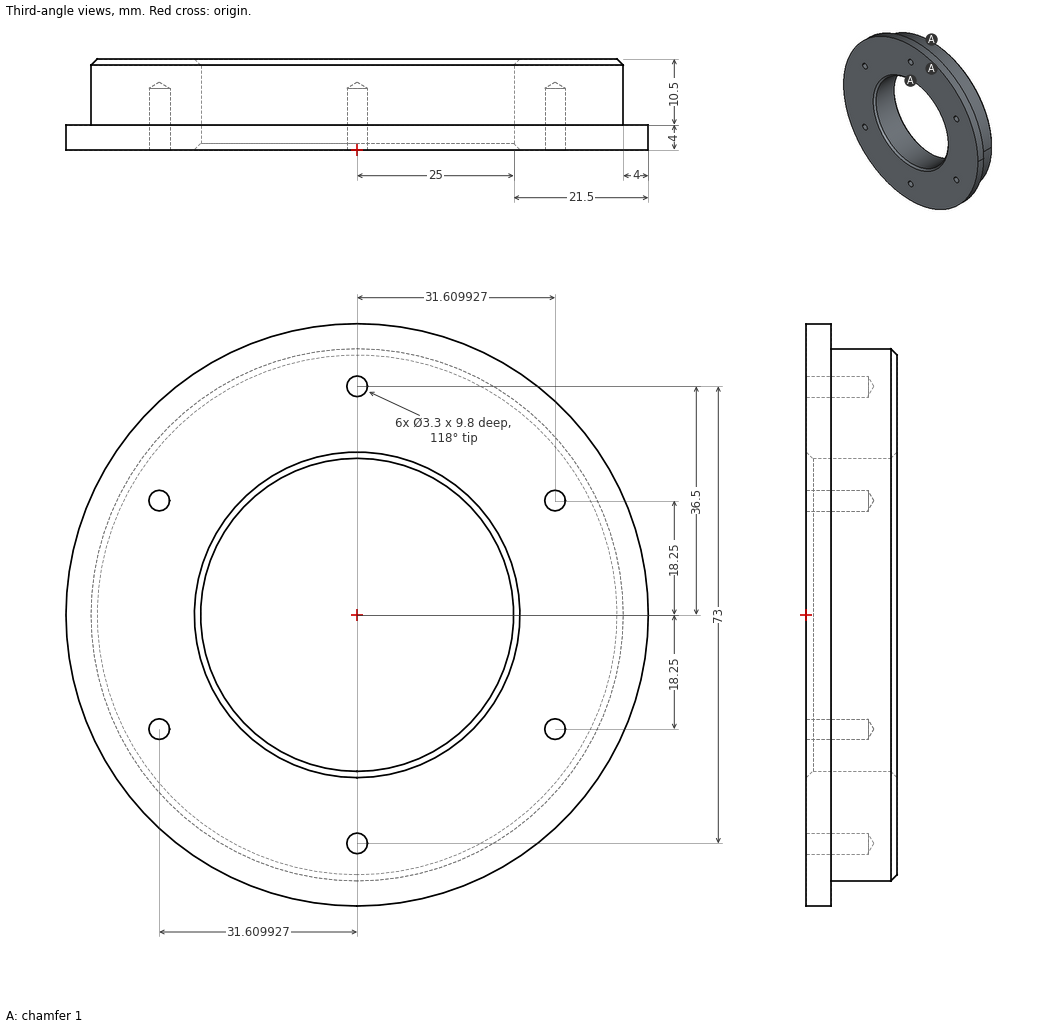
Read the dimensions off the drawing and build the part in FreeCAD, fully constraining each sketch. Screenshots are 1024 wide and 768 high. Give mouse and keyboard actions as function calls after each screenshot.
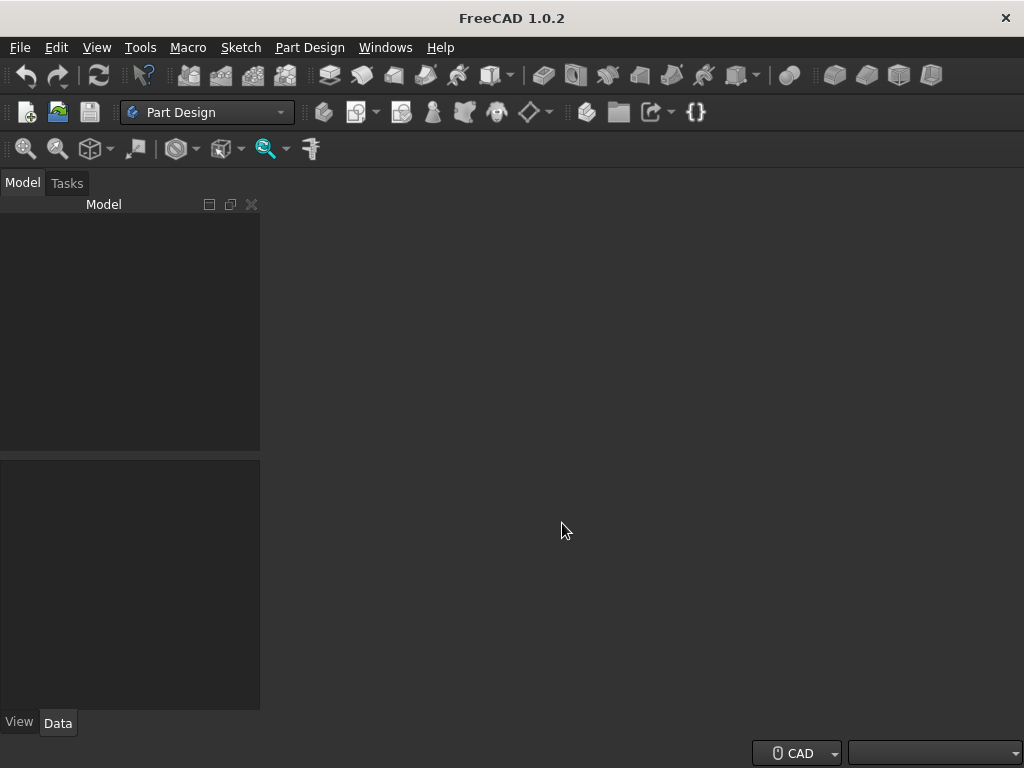
click(26, 112)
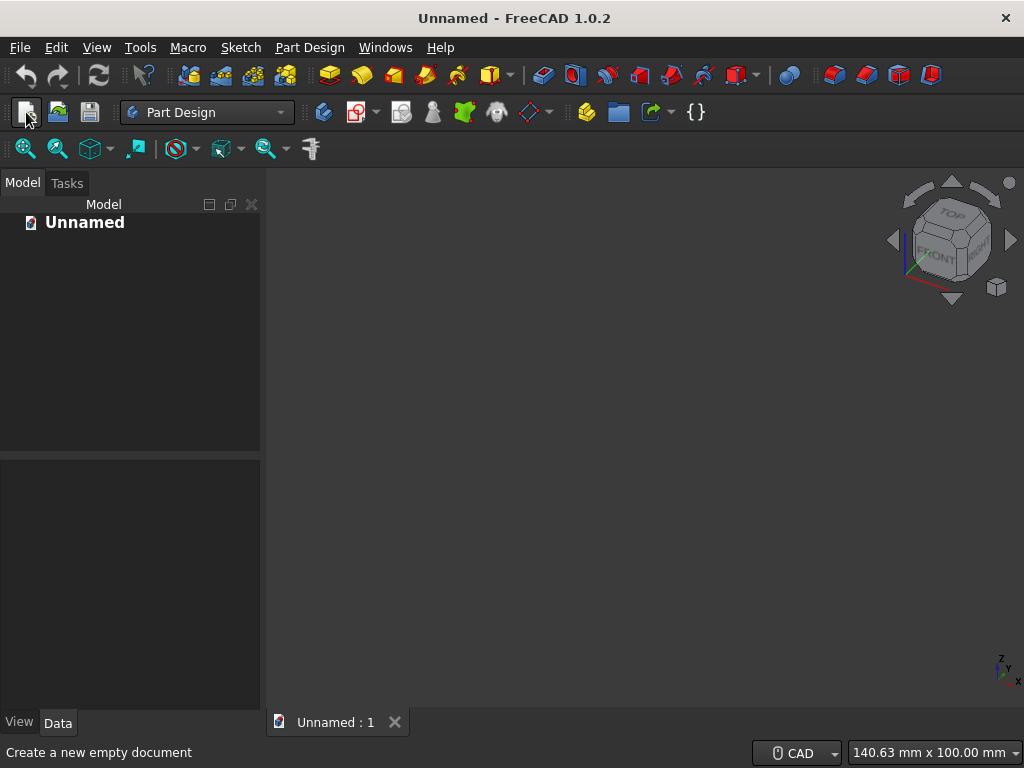
click(356, 112)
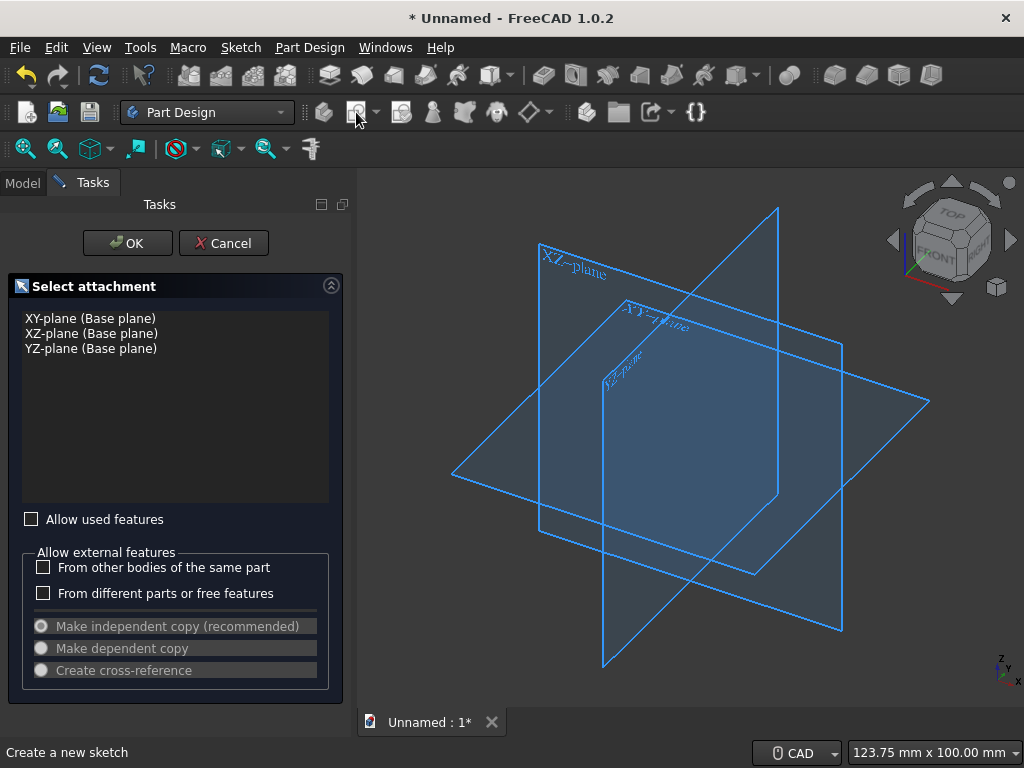
click(82, 318)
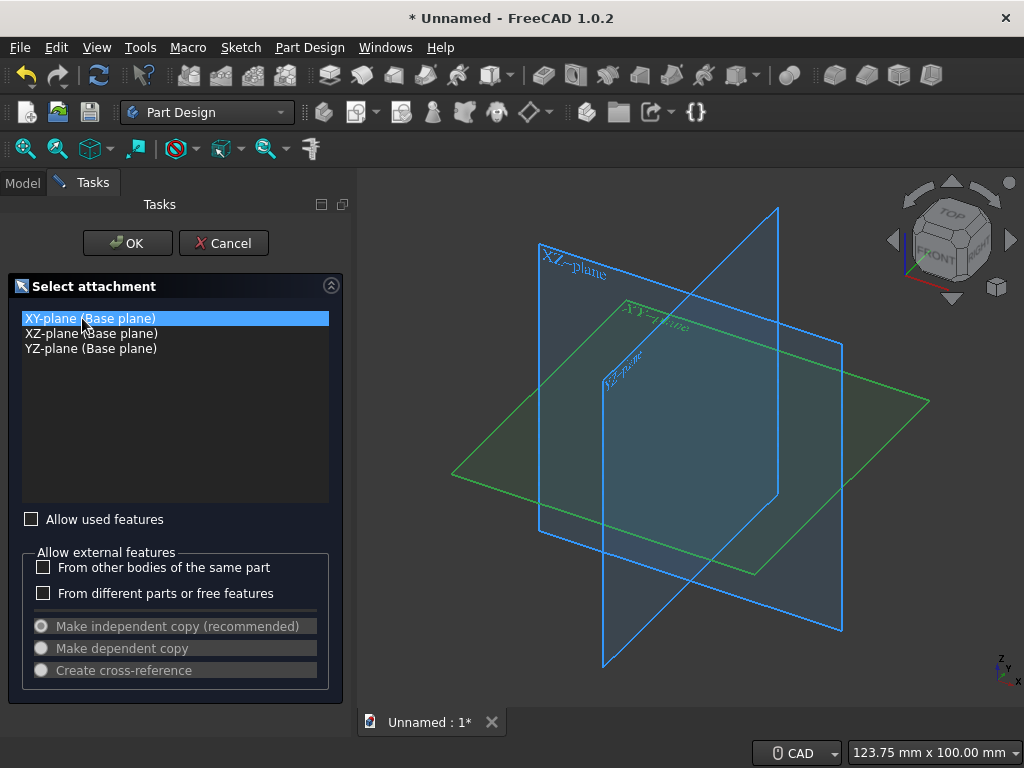
click(128, 243)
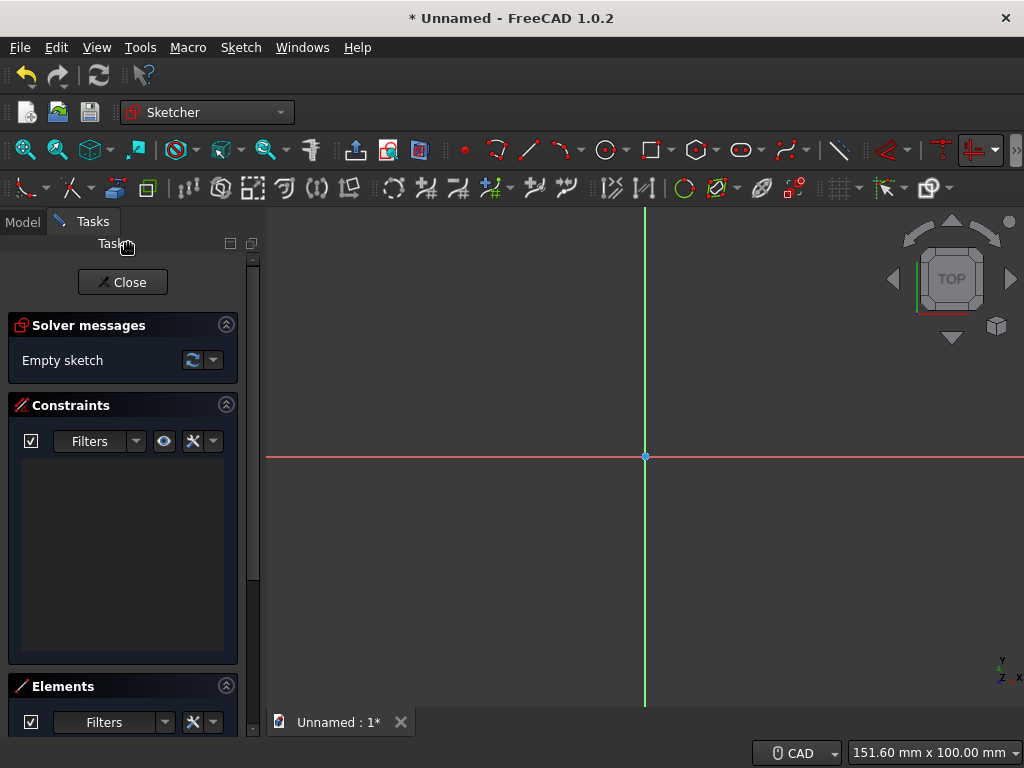
scroll(576, 457, down, 5)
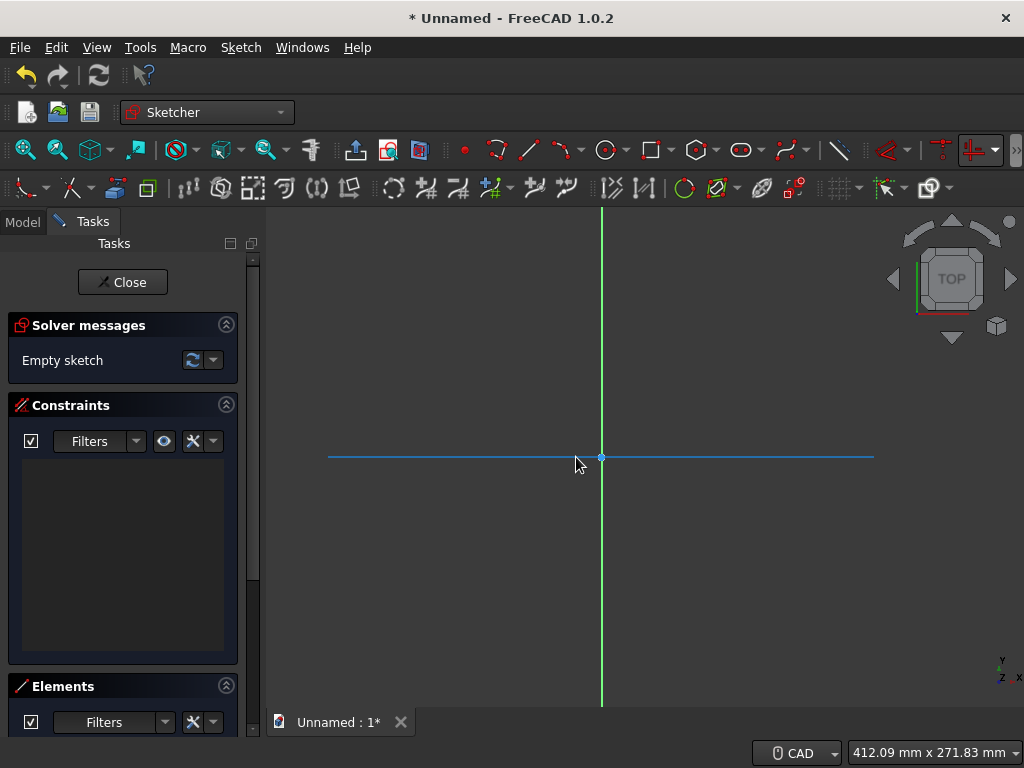
scroll(662, 441, up, 8)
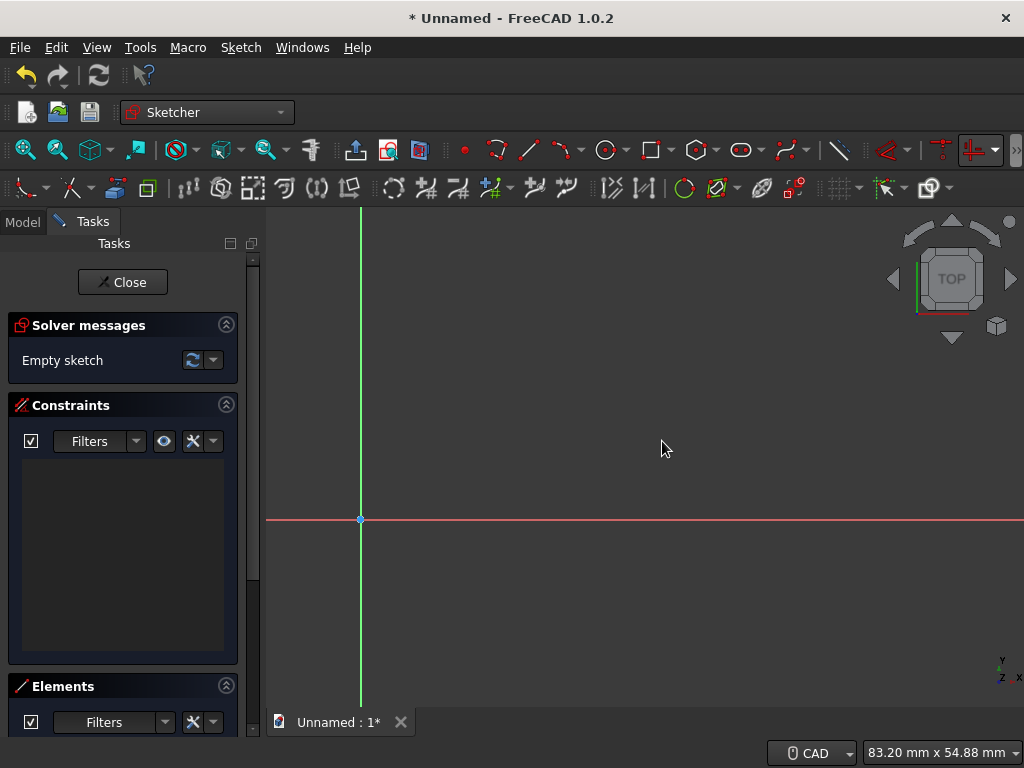
click(498, 150)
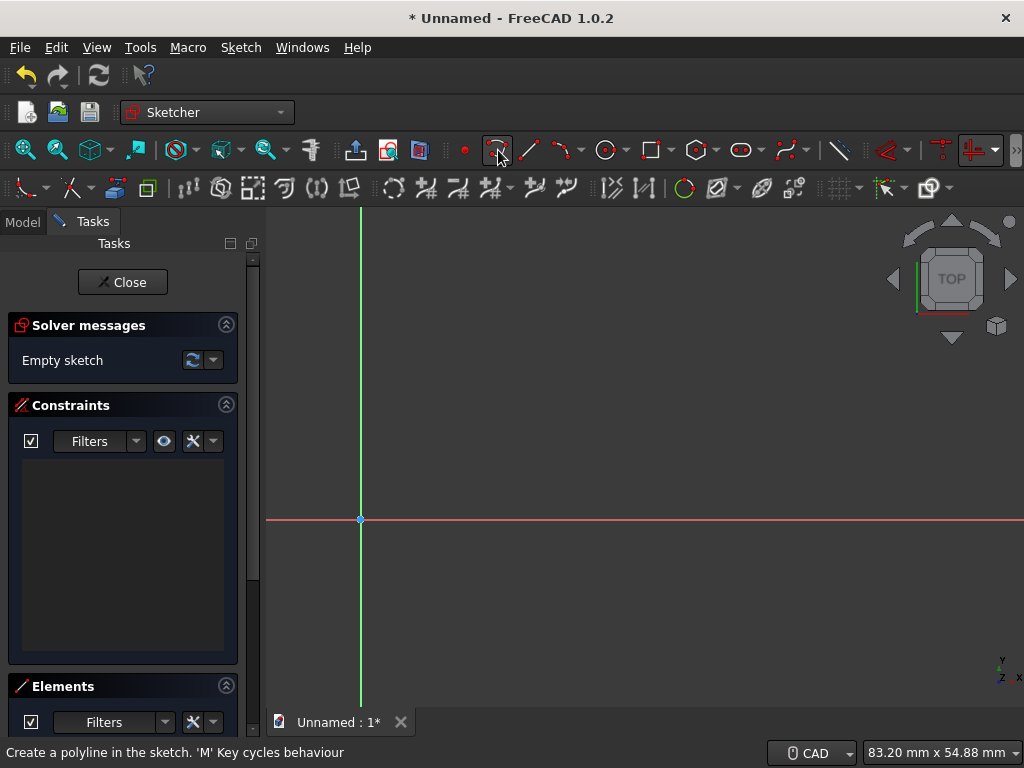
click(589, 520)
click(785, 511)
click(785, 484)
click(748, 484)
click(748, 388)
click(589, 388)
click(589, 520)
key(Escape)
key(Escape)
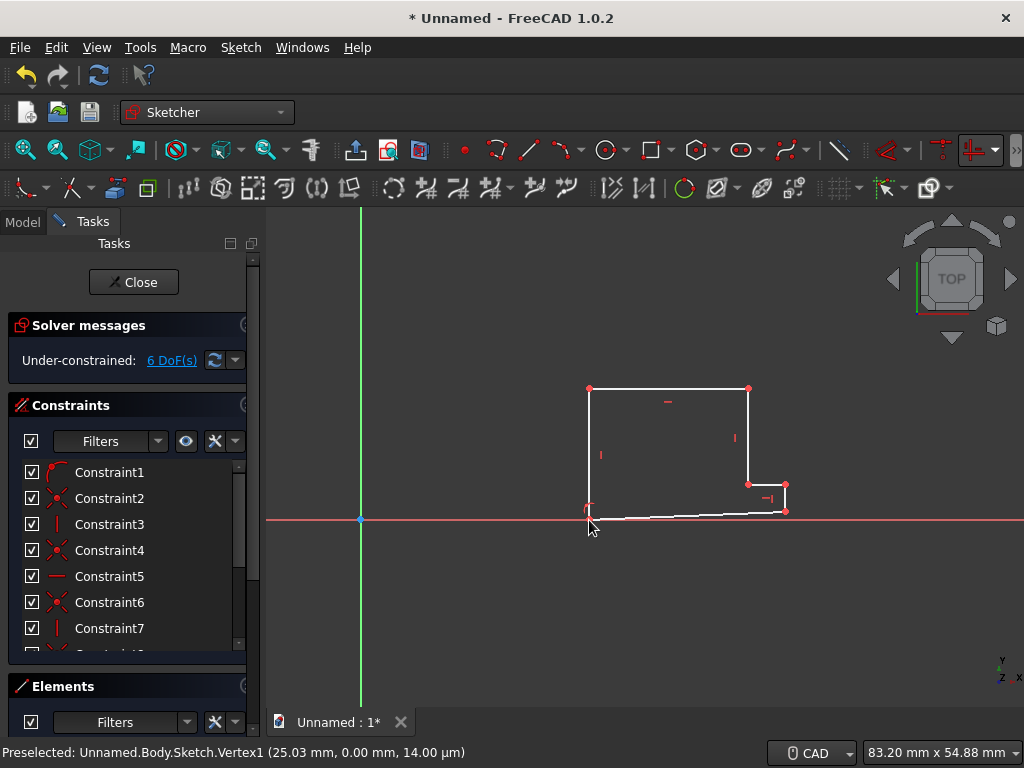
click(648, 518)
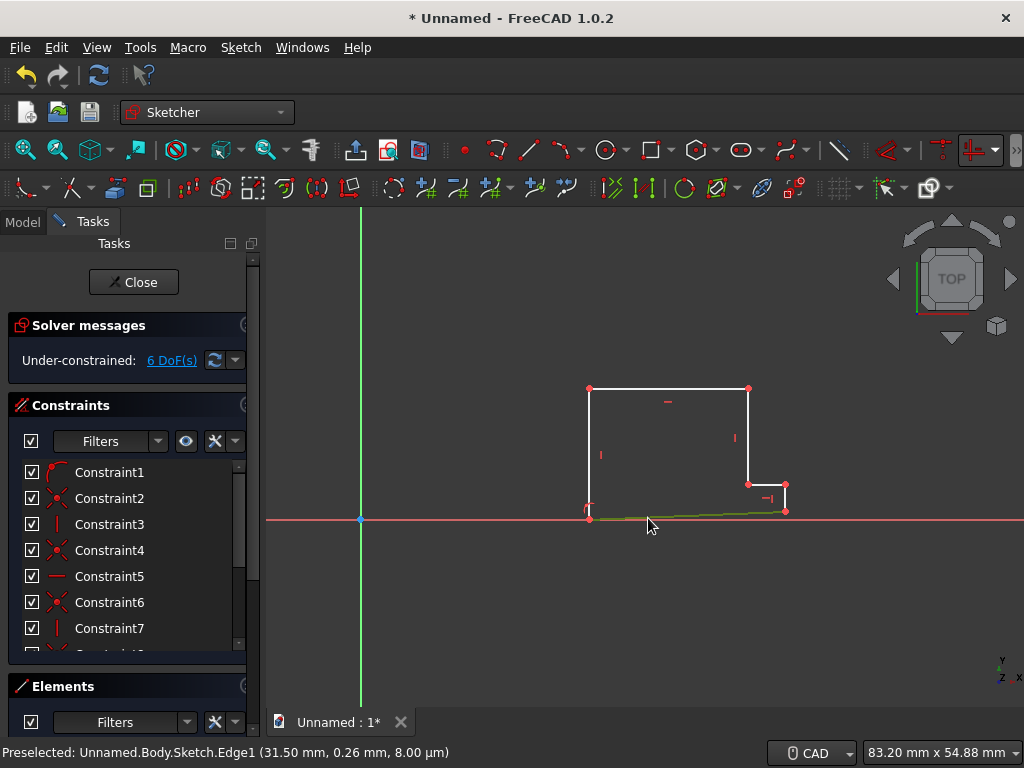
click(998, 150)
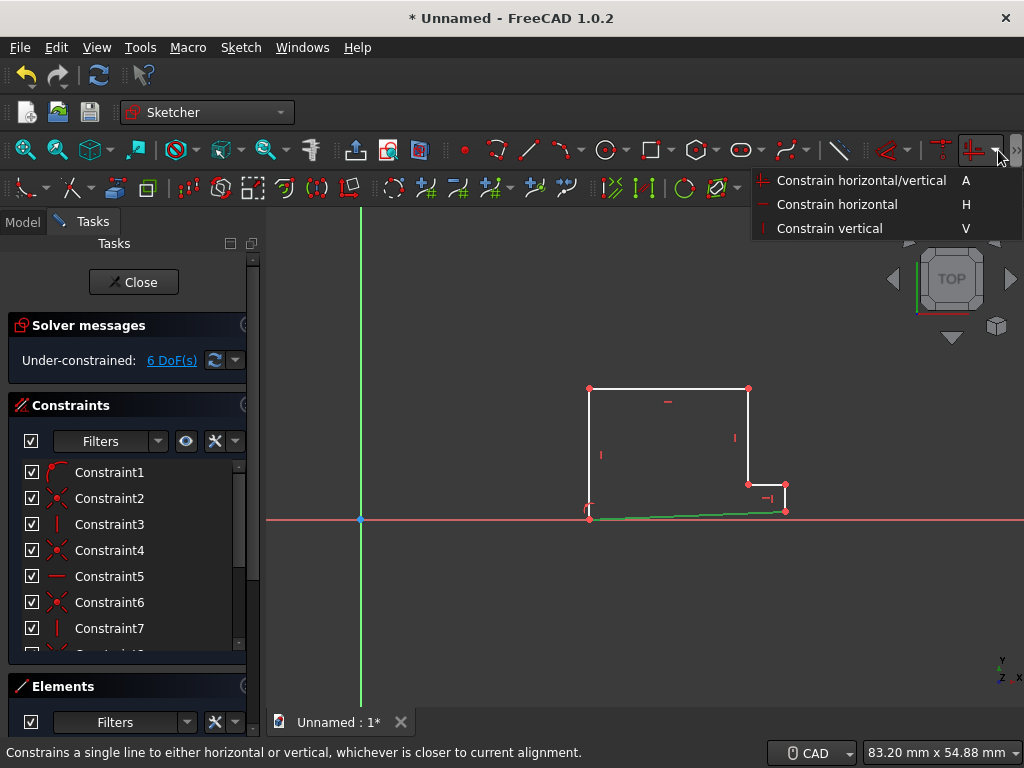
click(887, 204)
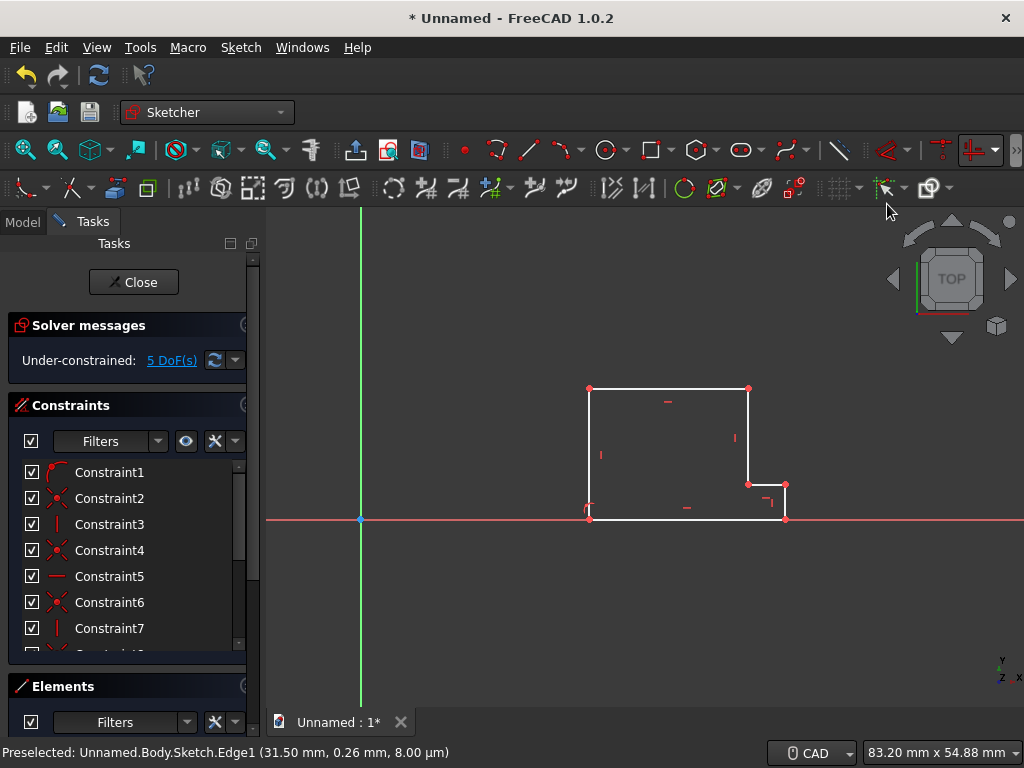
key(d)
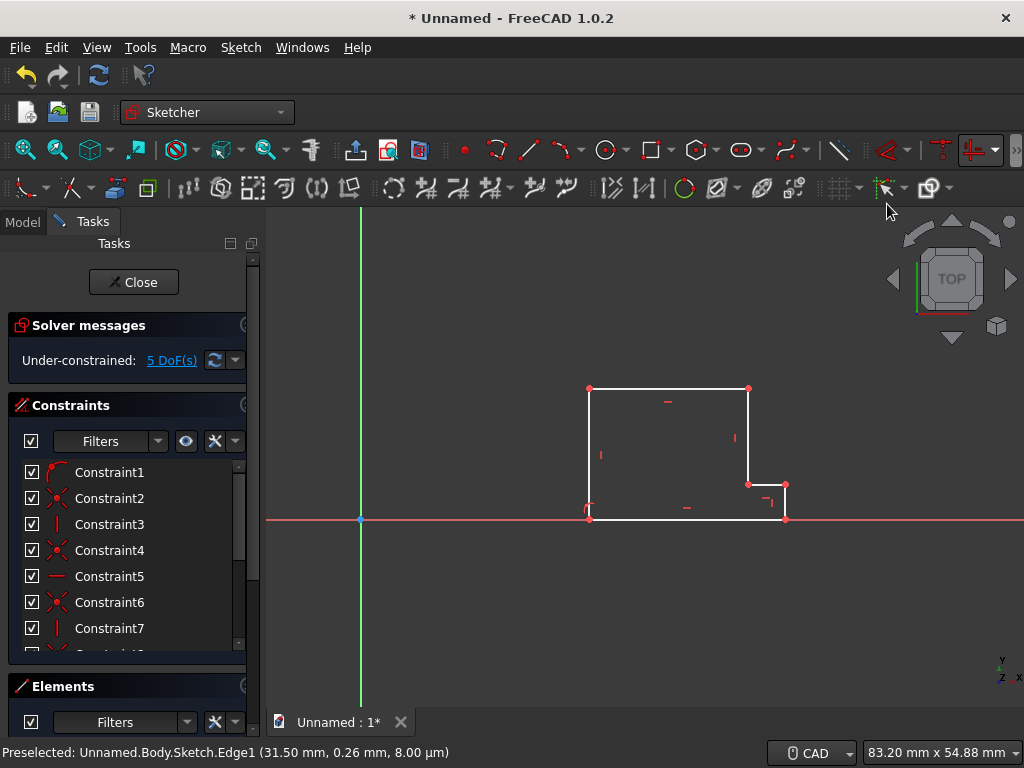
scroll(785, 509, up, 2)